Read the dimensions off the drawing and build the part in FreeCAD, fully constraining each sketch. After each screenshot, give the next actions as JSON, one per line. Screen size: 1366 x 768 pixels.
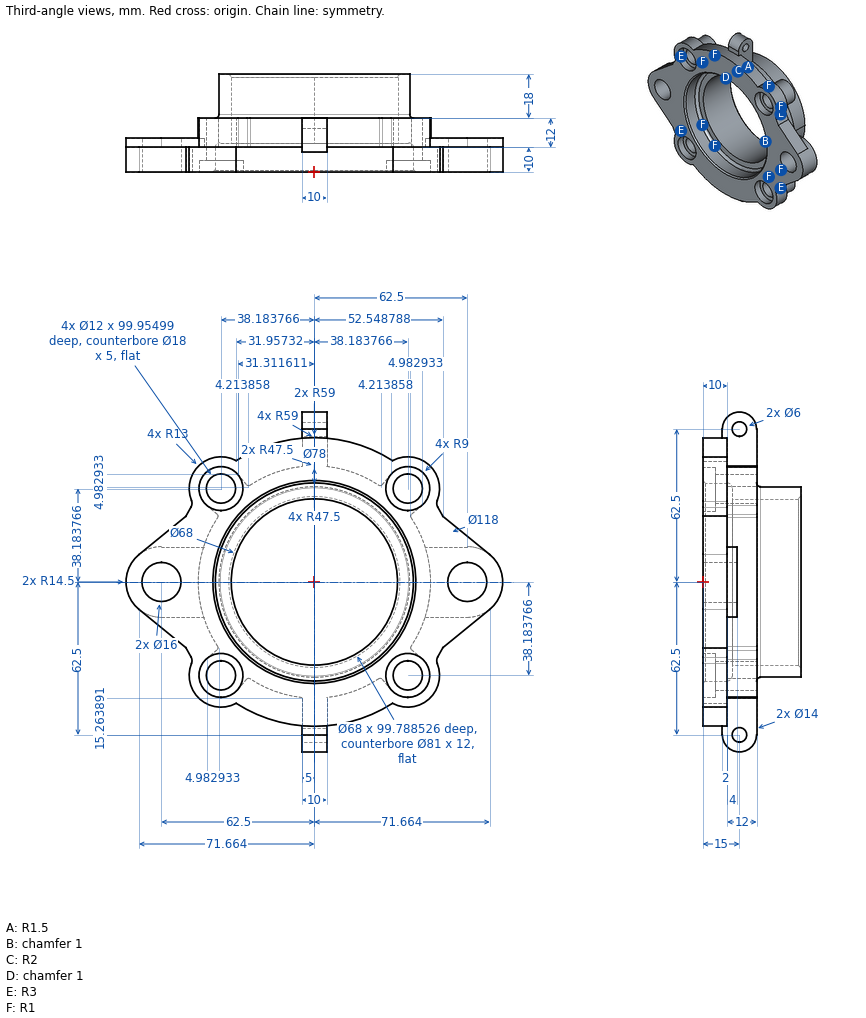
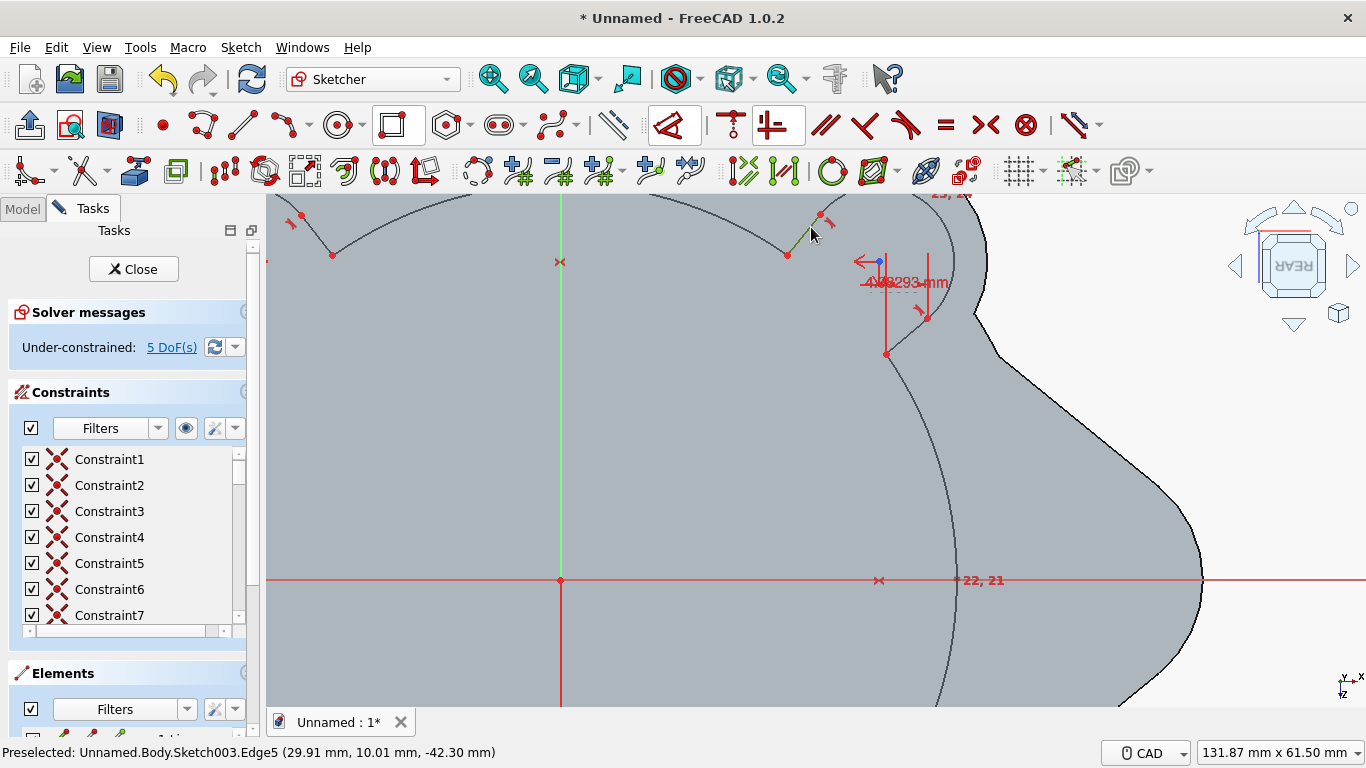
{"action": "left_click", "coordinate": [696, 126]}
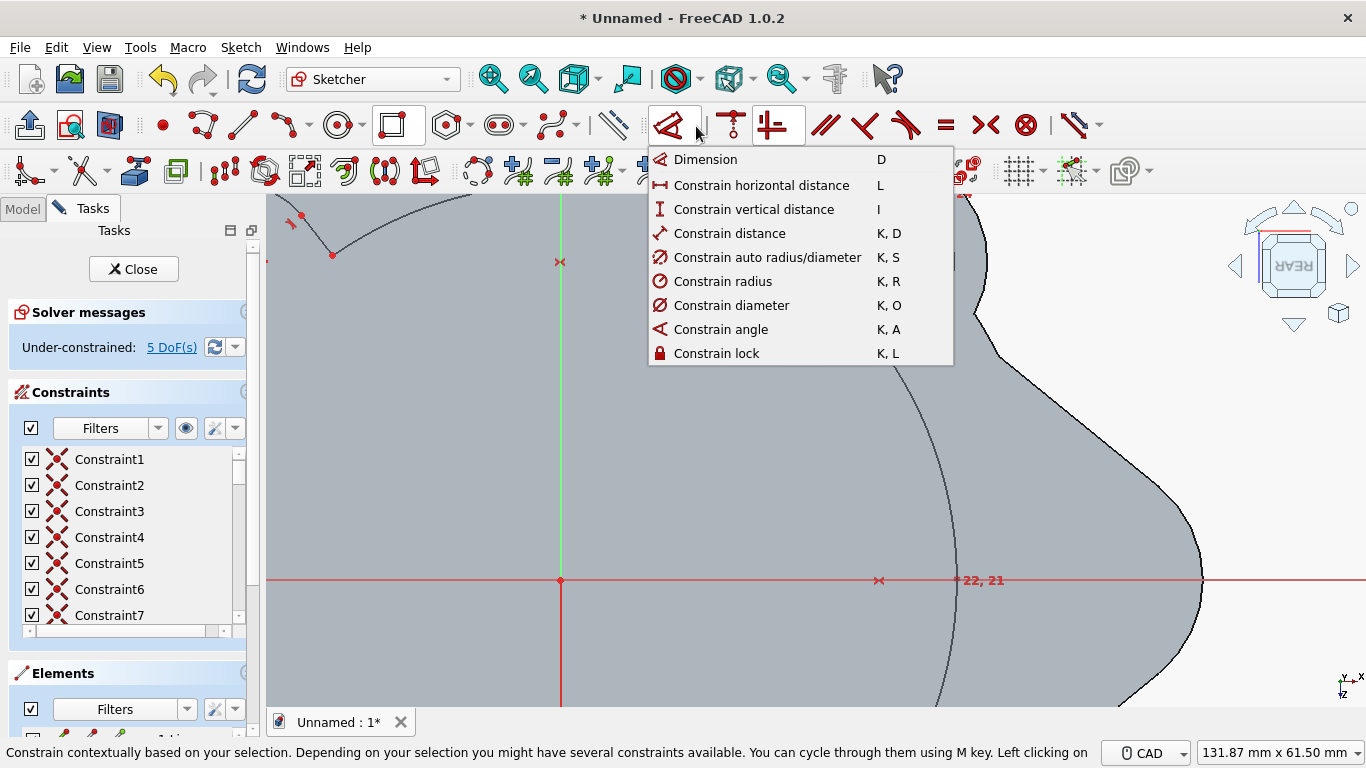
{"action": "left_click", "coordinate": [801, 185]}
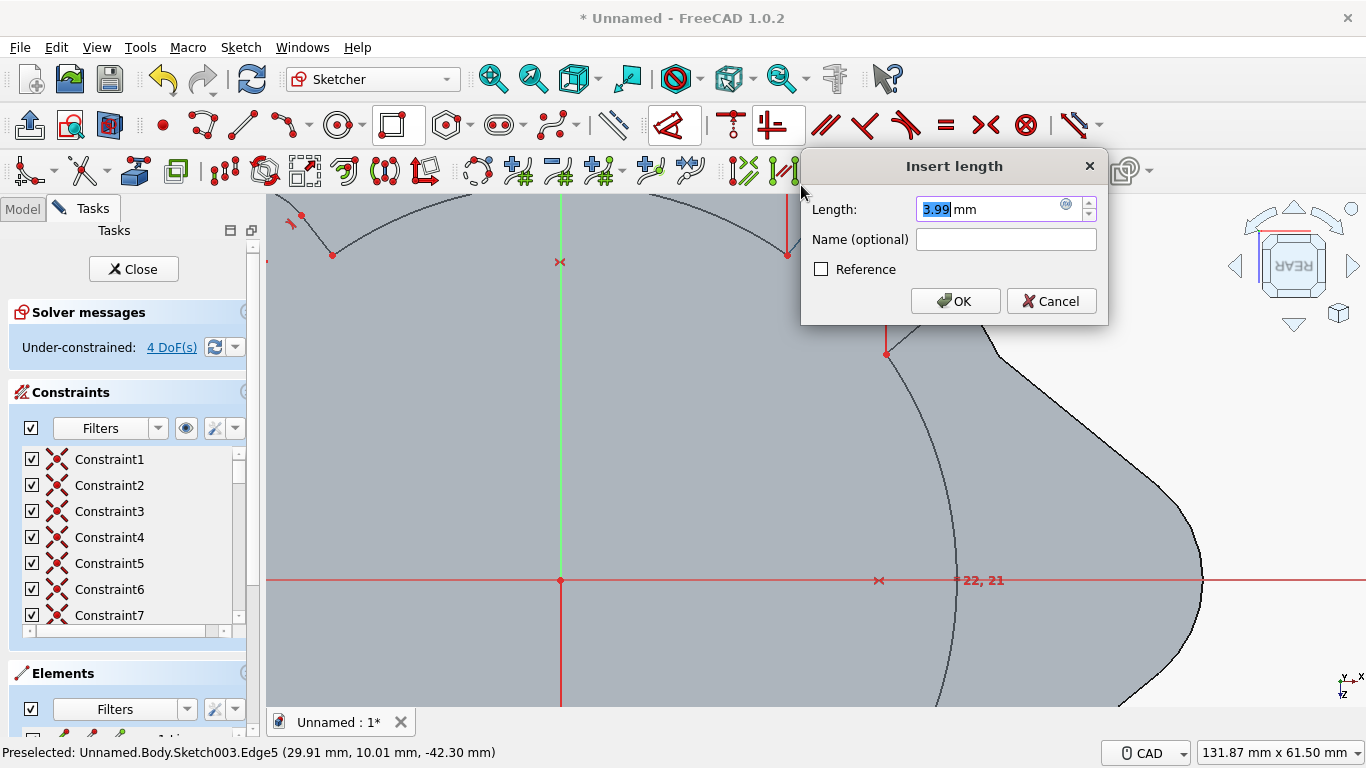
{"action": "type", "text": "4.213858"}
{"action": "key", "text": "Return"}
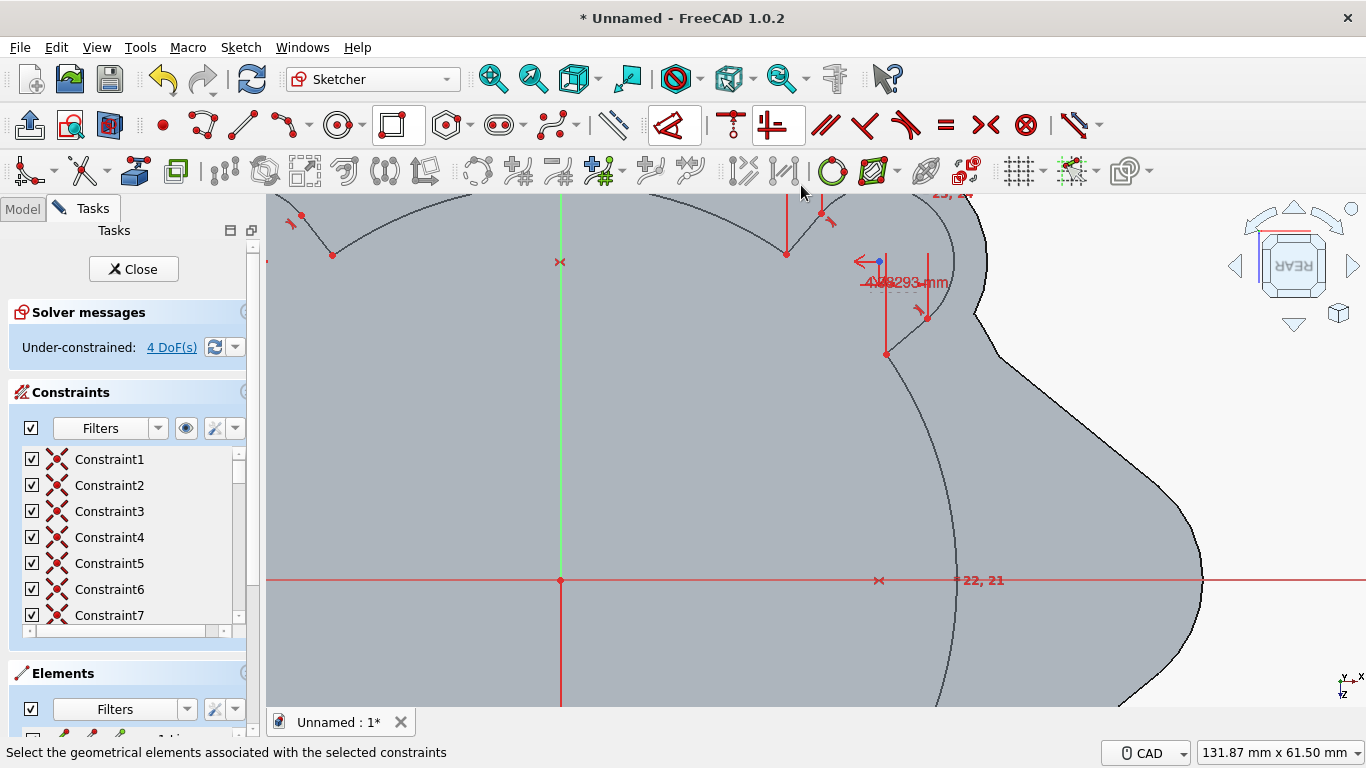
{"action": "left_click", "coordinate": [324, 244]}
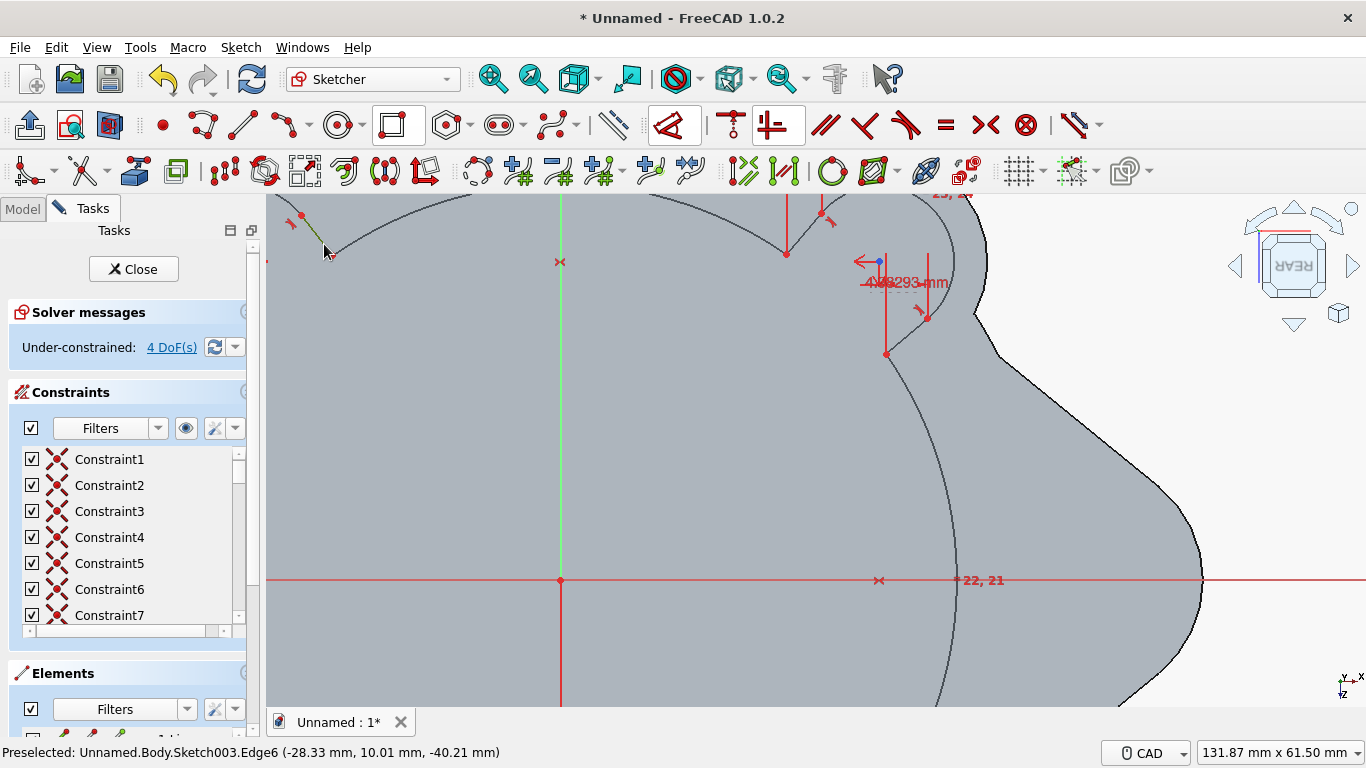
{"action": "left_click", "coordinate": [696, 126]}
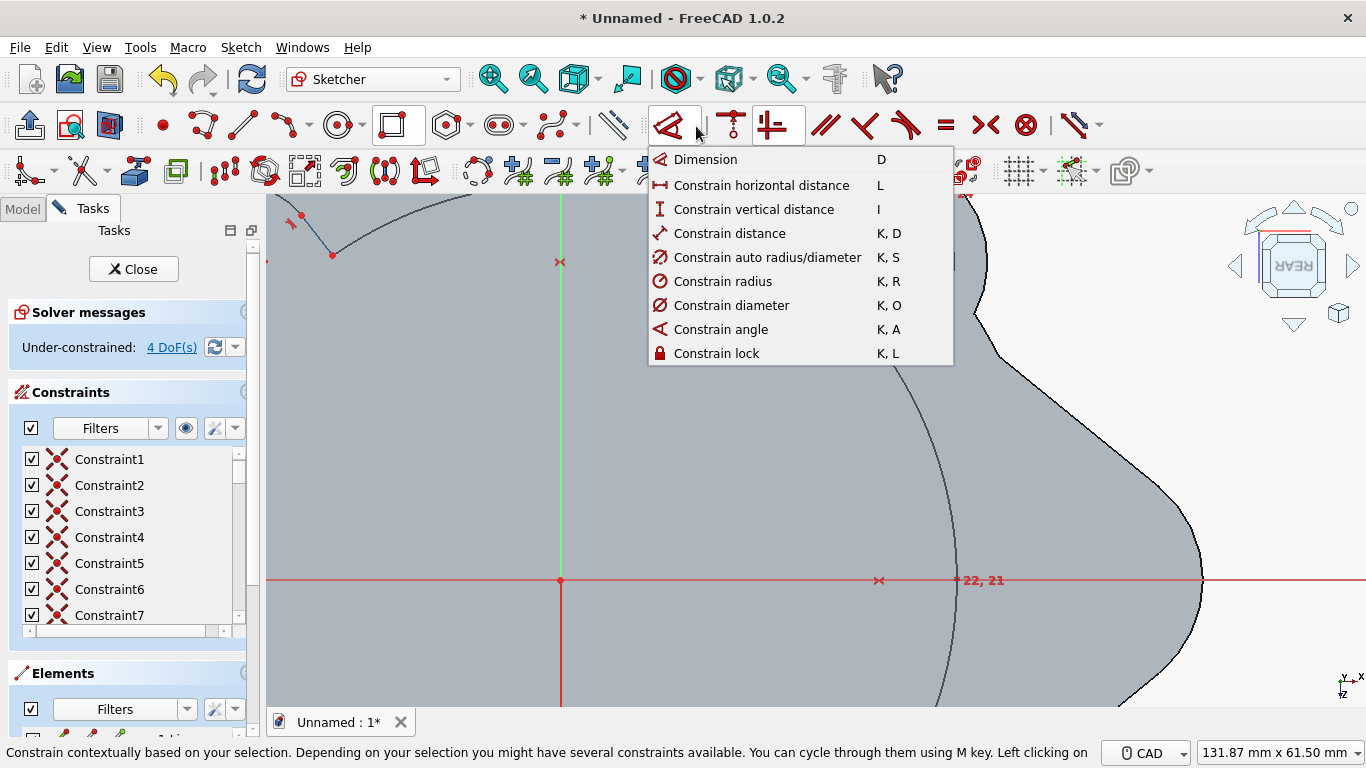
{"action": "left_click", "coordinate": [801, 185]}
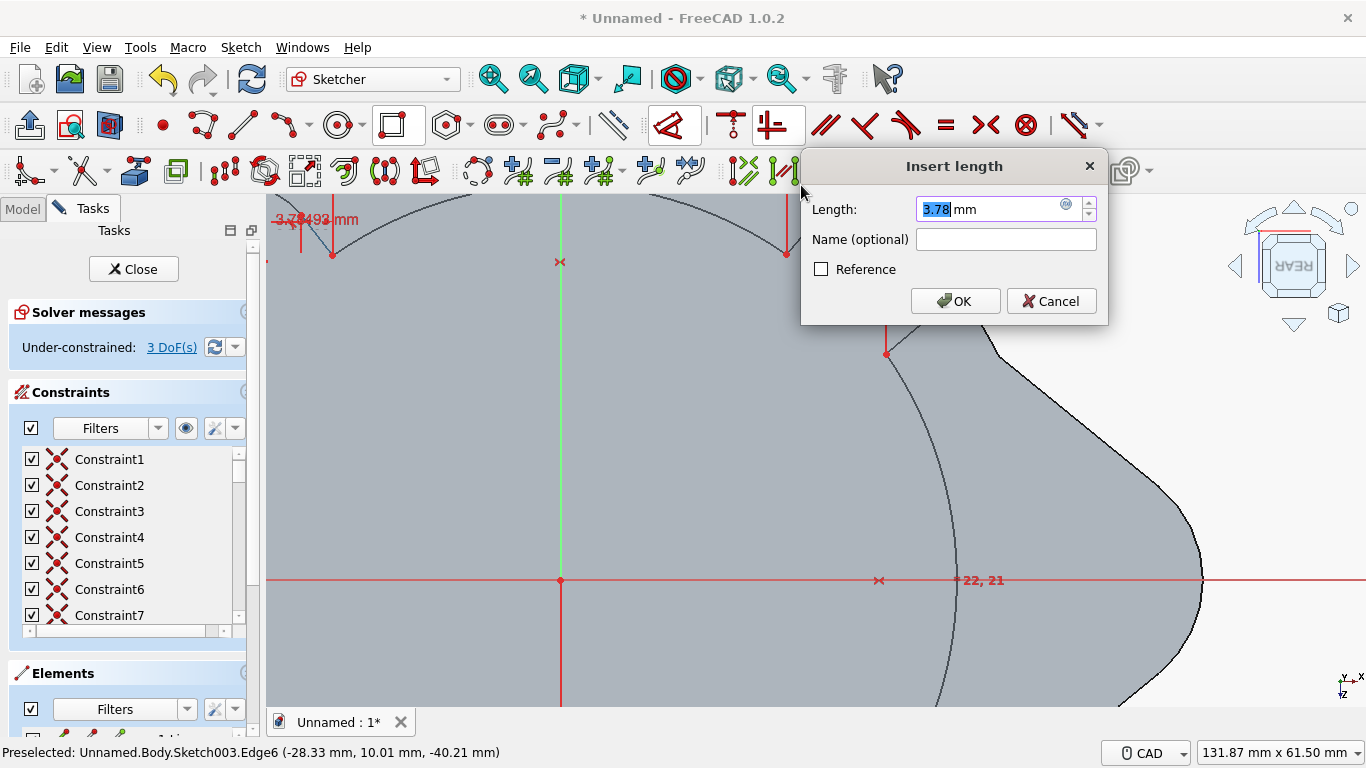
{"action": "type", "text": "4.213858"}
{"action": "key", "text": "Return"}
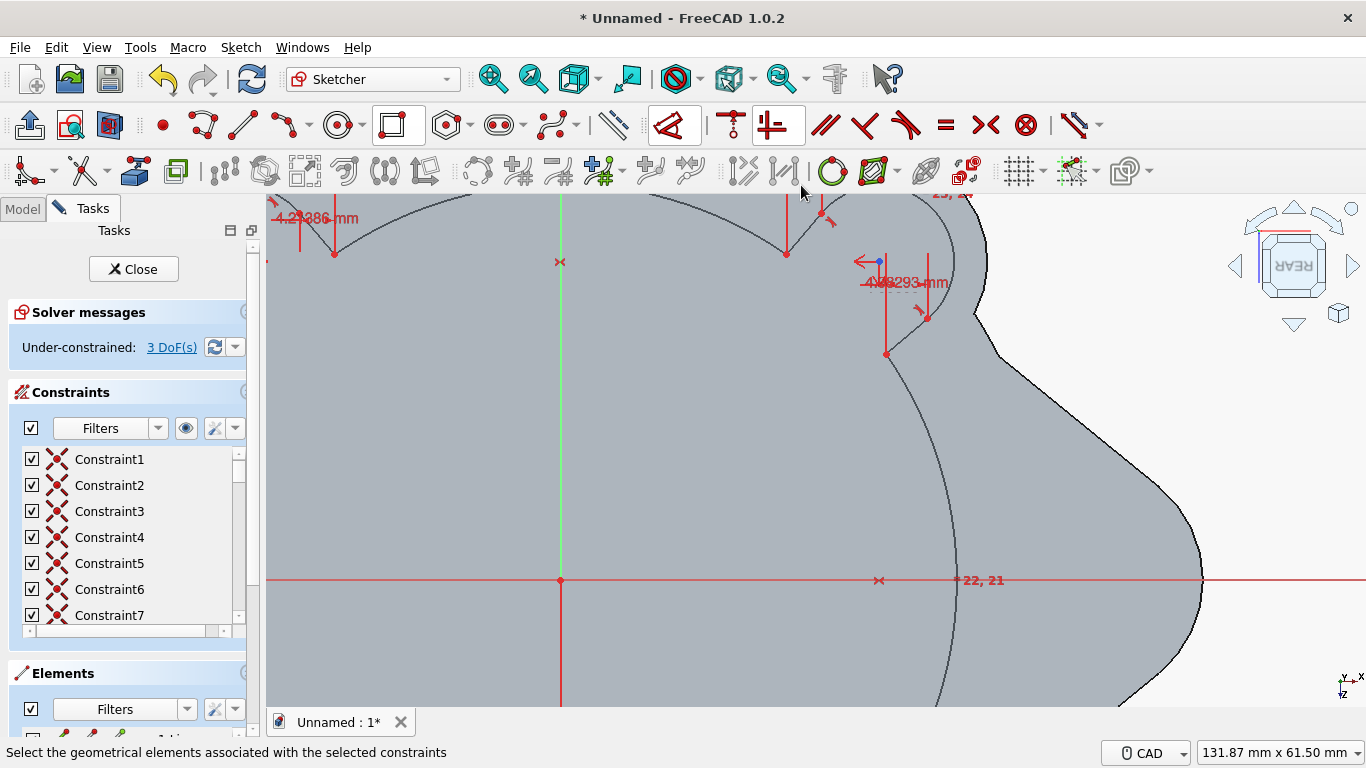
{"action": "scroll", "coordinate": [900, 345], "scroll_direction": "down", "scroll_amount": 4}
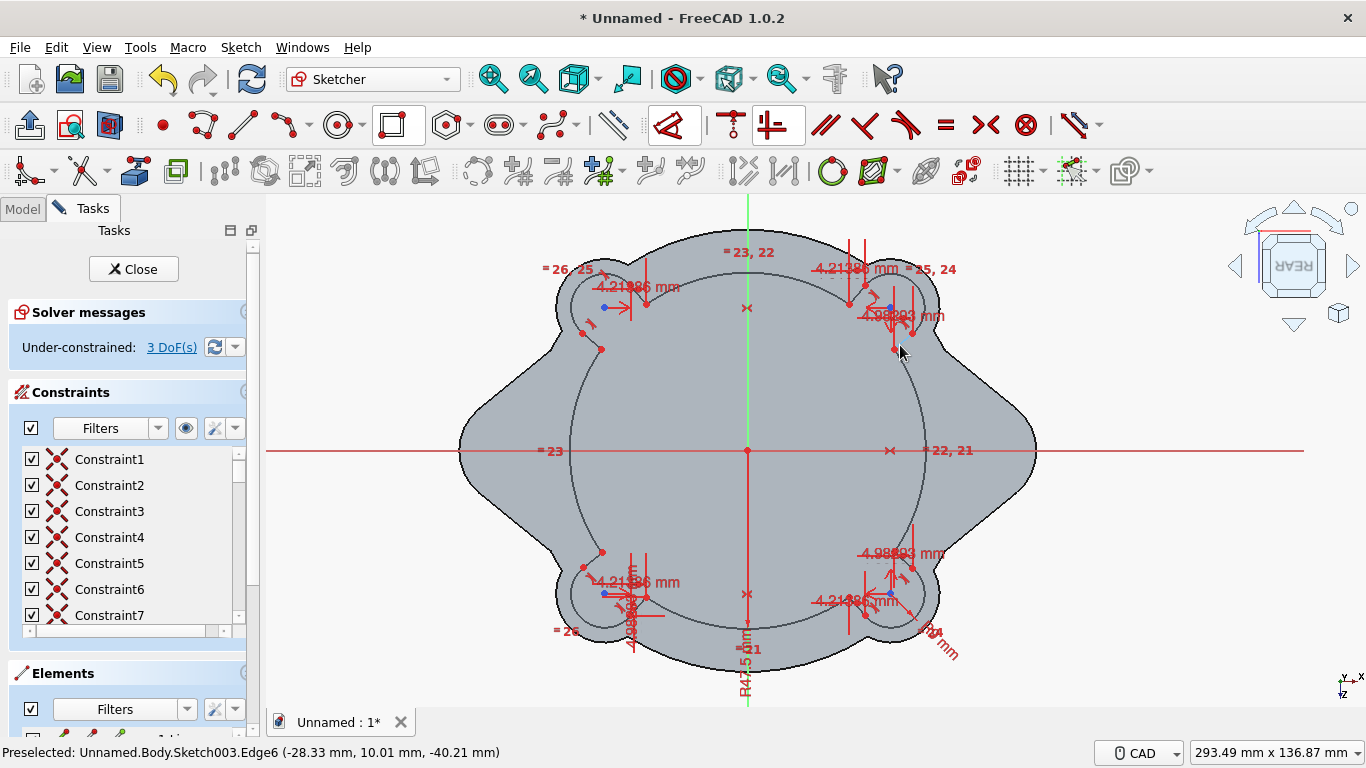
{"action": "scroll", "coordinate": [589, 338], "scroll_direction": "up", "scroll_amount": 4}